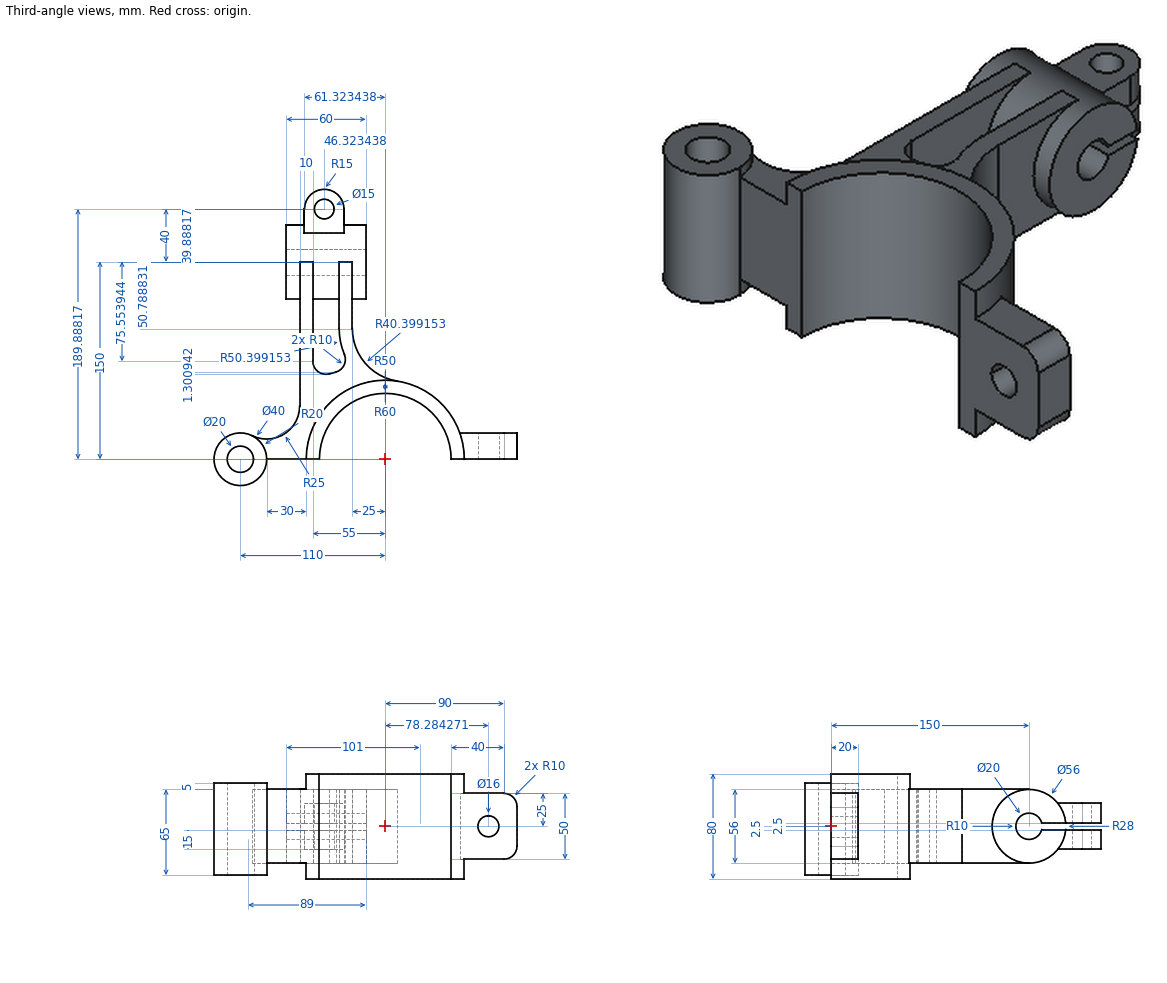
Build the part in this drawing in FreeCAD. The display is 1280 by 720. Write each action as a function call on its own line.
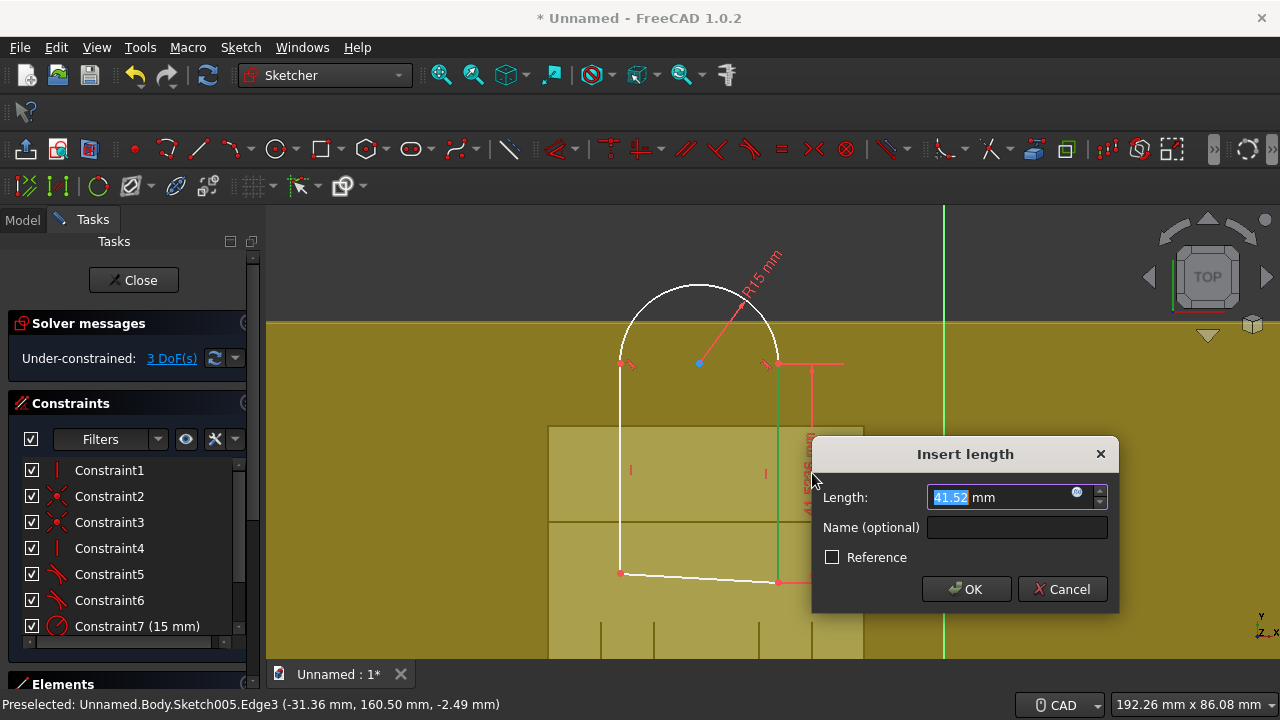
text(40)
key(Return)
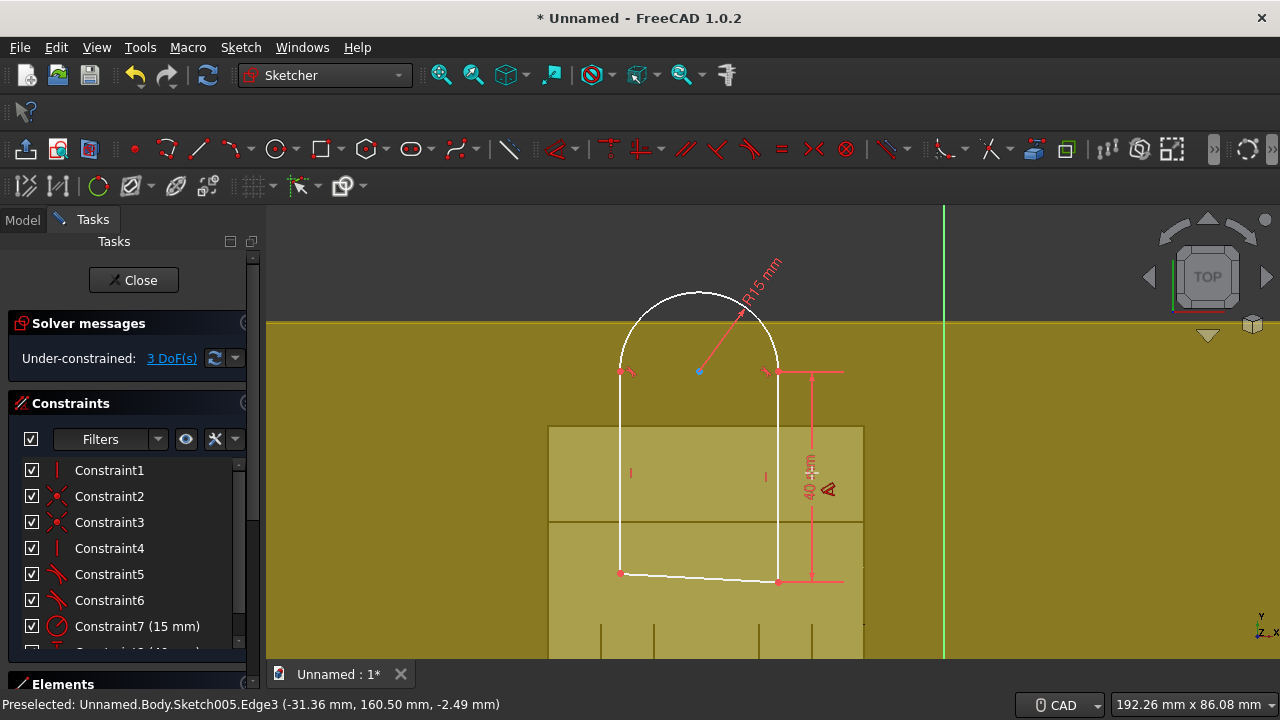
click(620, 574)
click(978, 603)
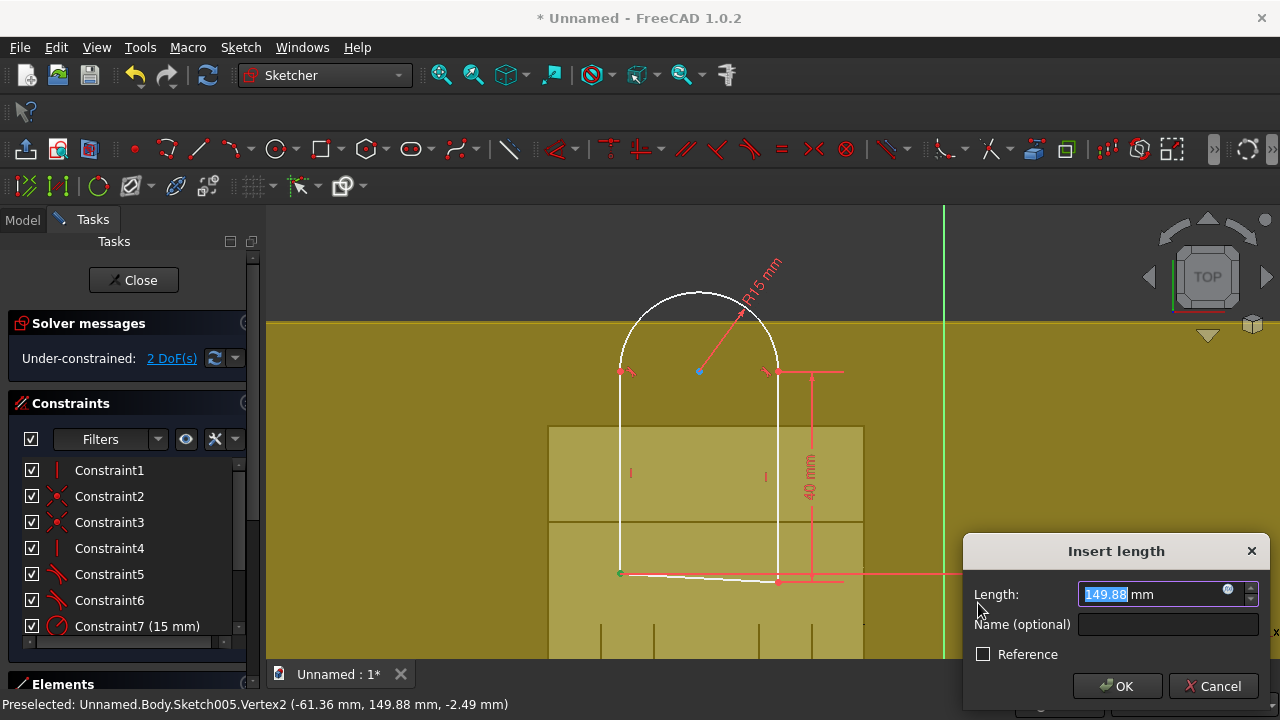
text(150)
key(Return)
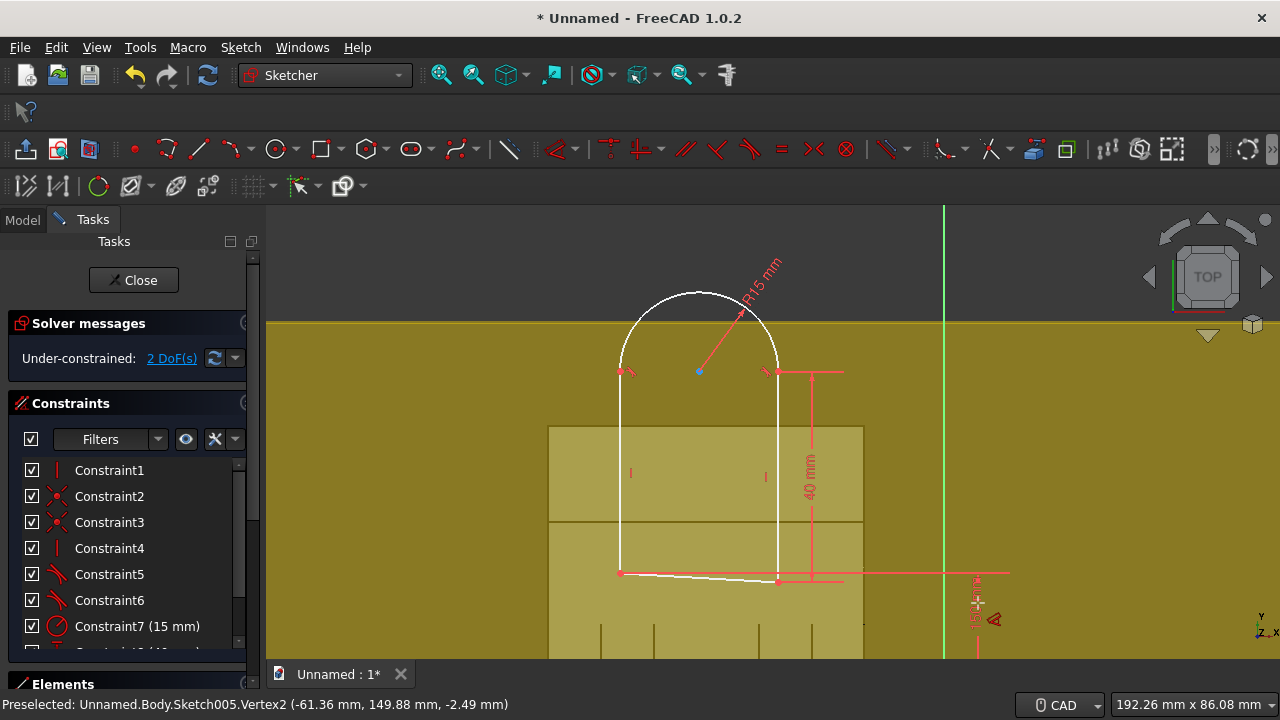
click(620, 432)
click(586, 472)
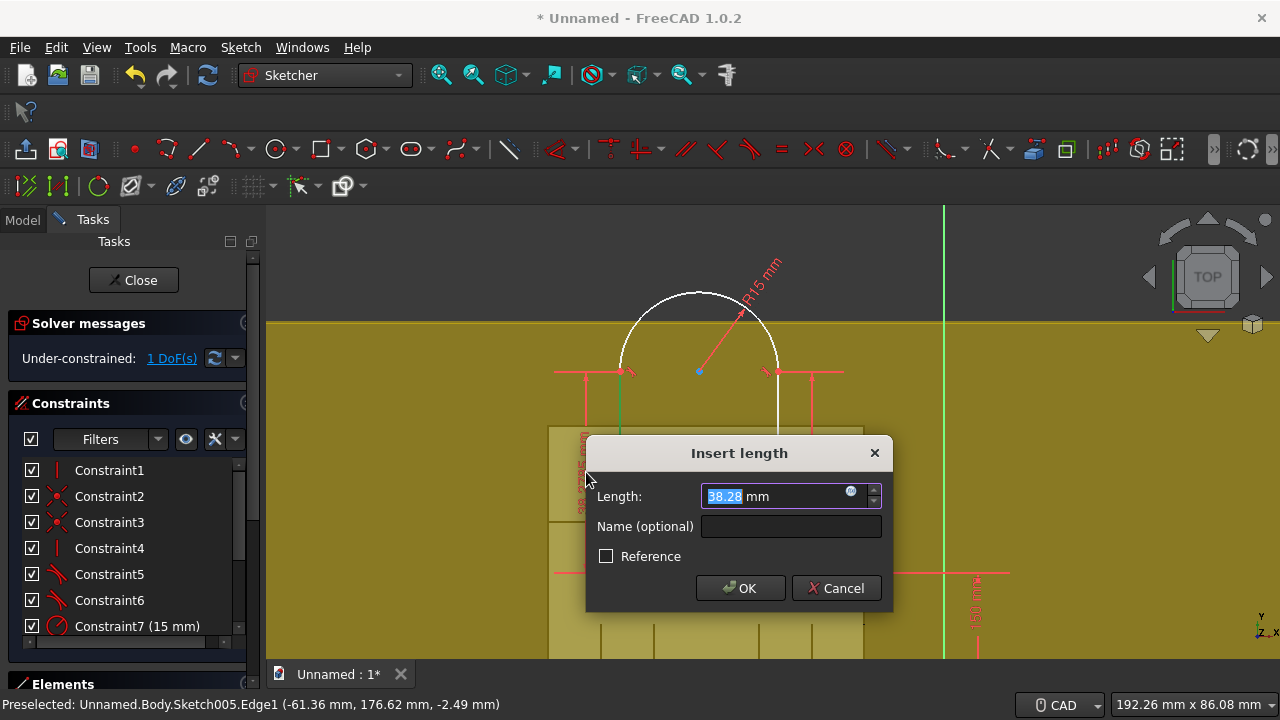
text(39.88817)
key(Return)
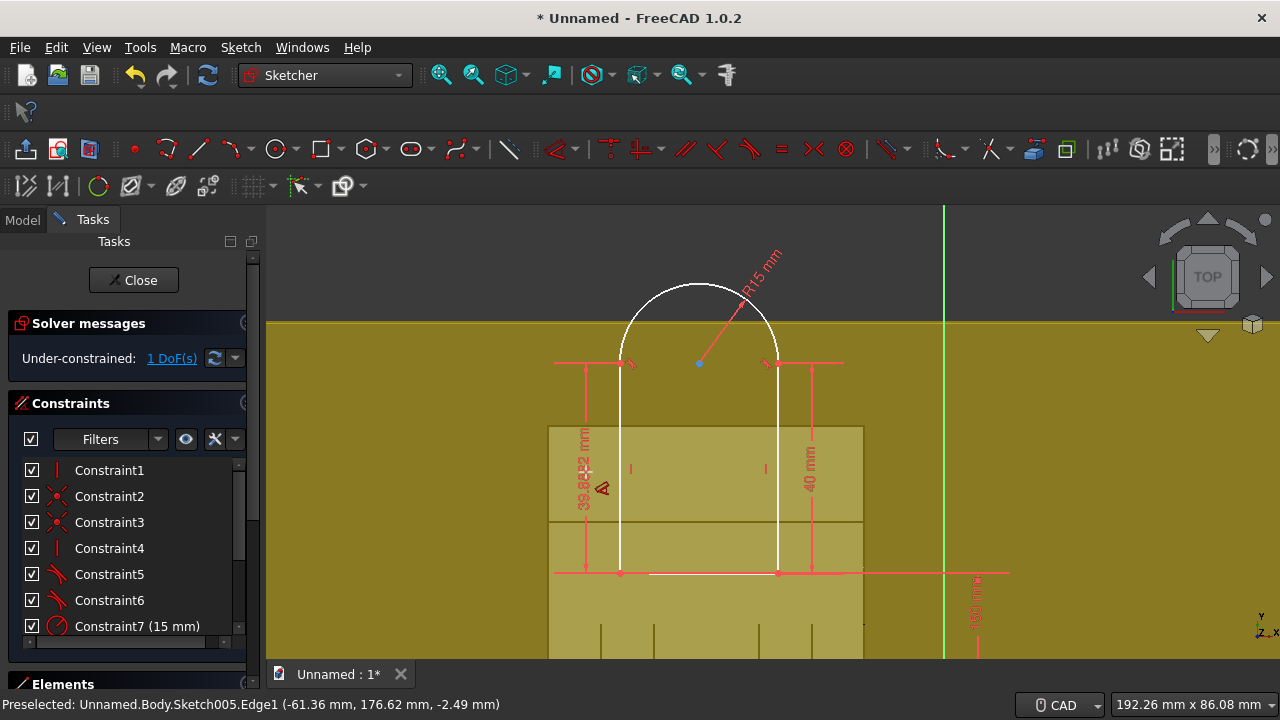
click(620, 363)
click(707, 329)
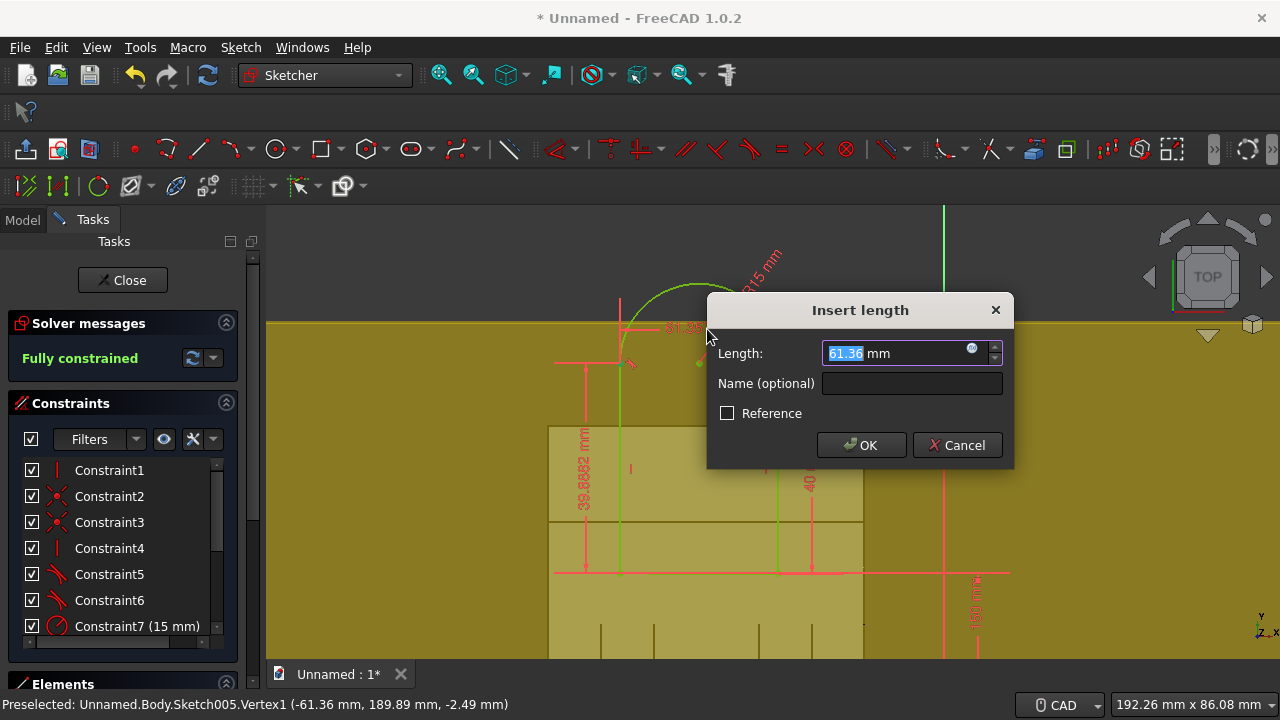
text(61.323438)
key(Return)
key(Escape)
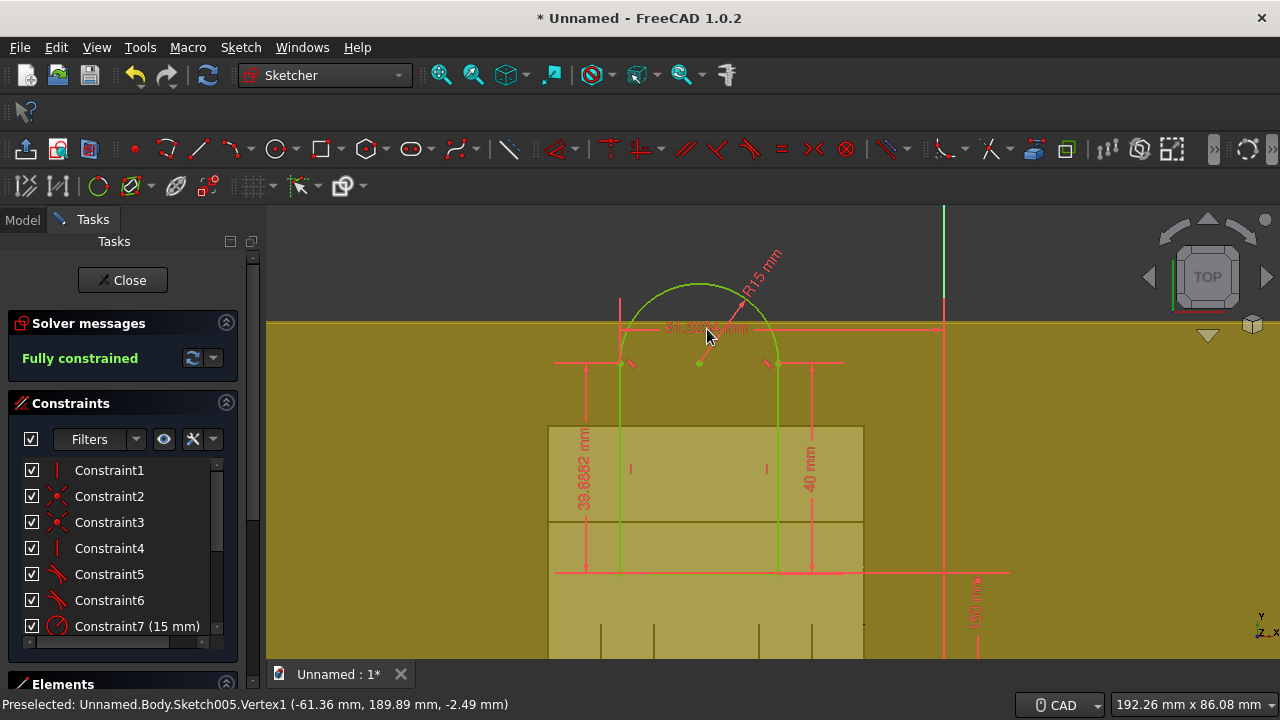
click(123, 280)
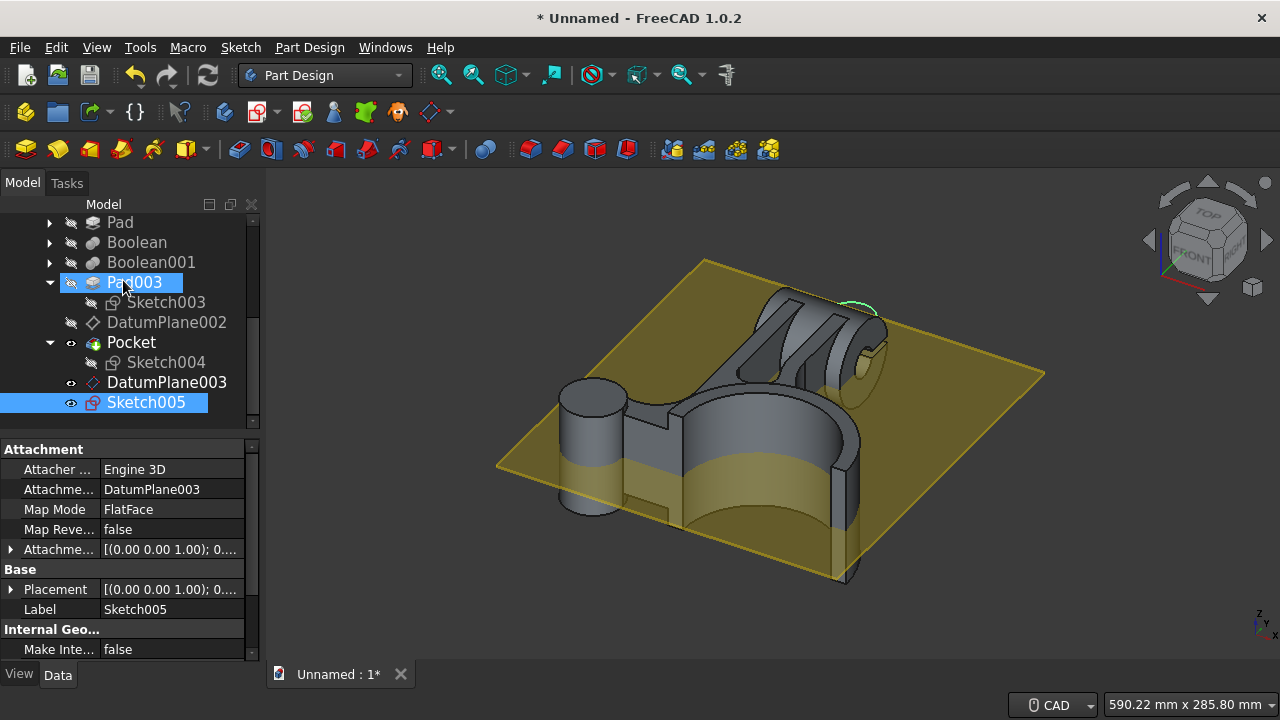
click(26, 150)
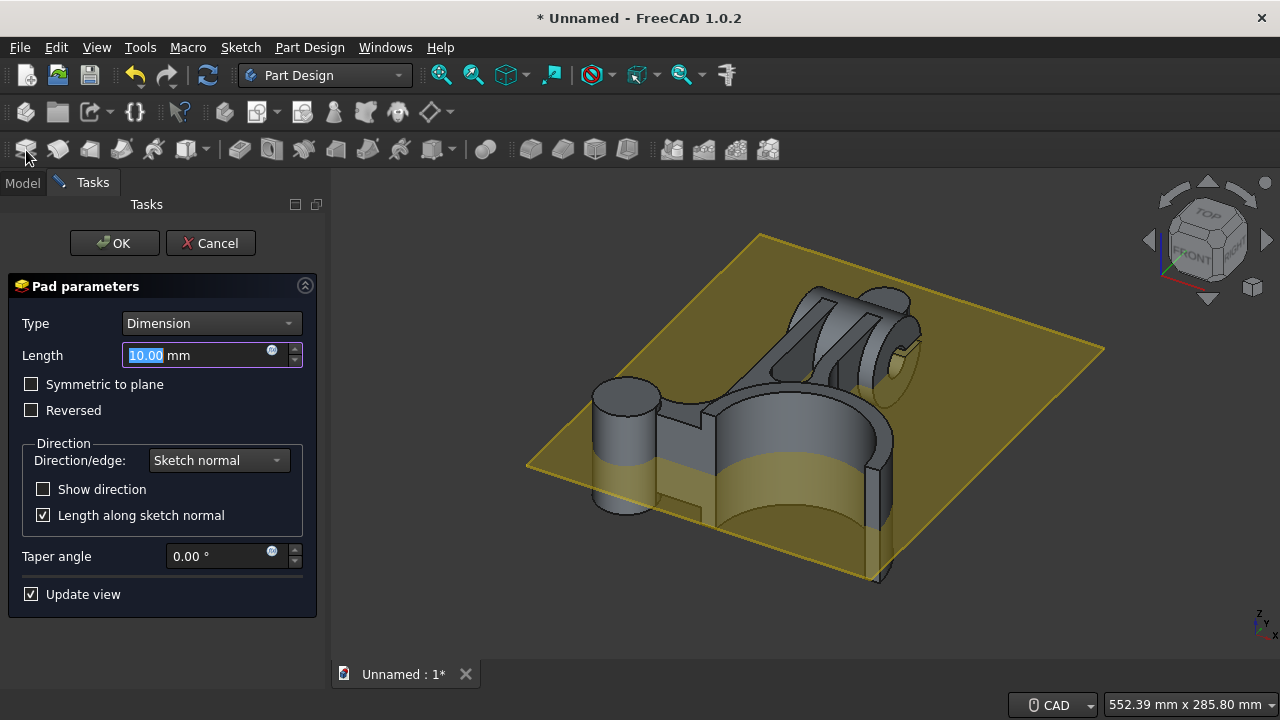
text(15)
key(Tab)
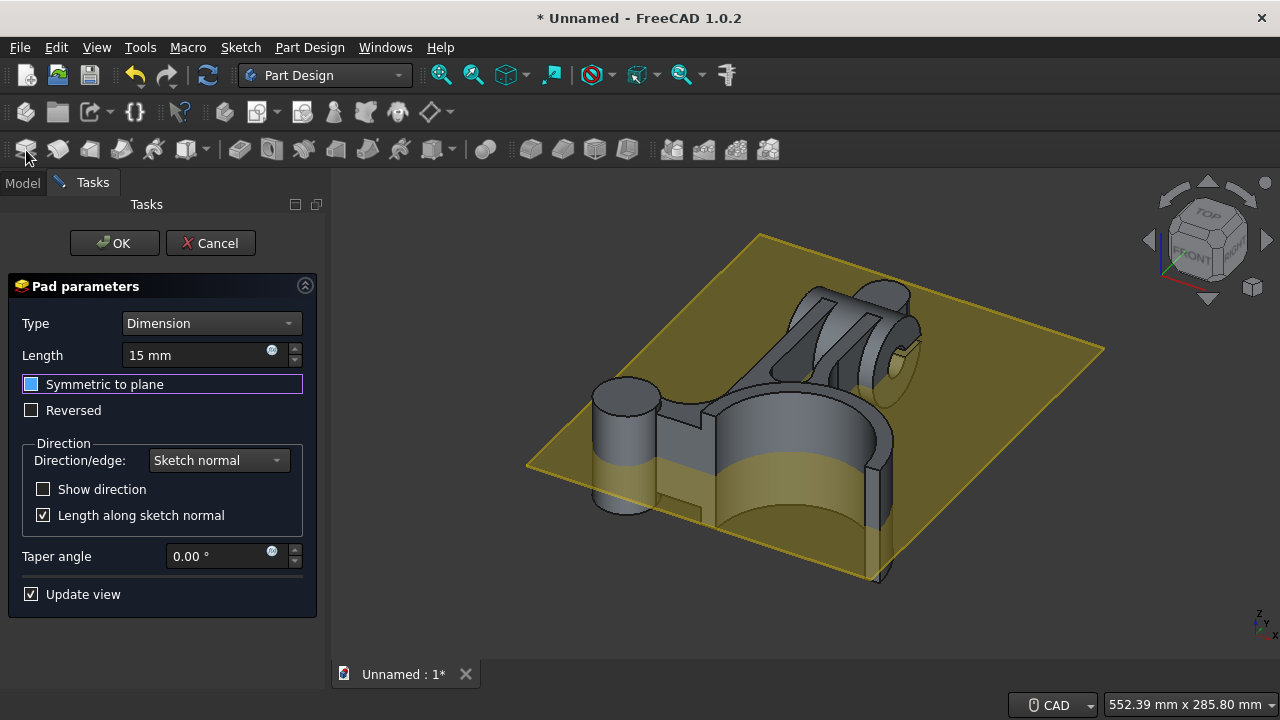
click(30, 410)